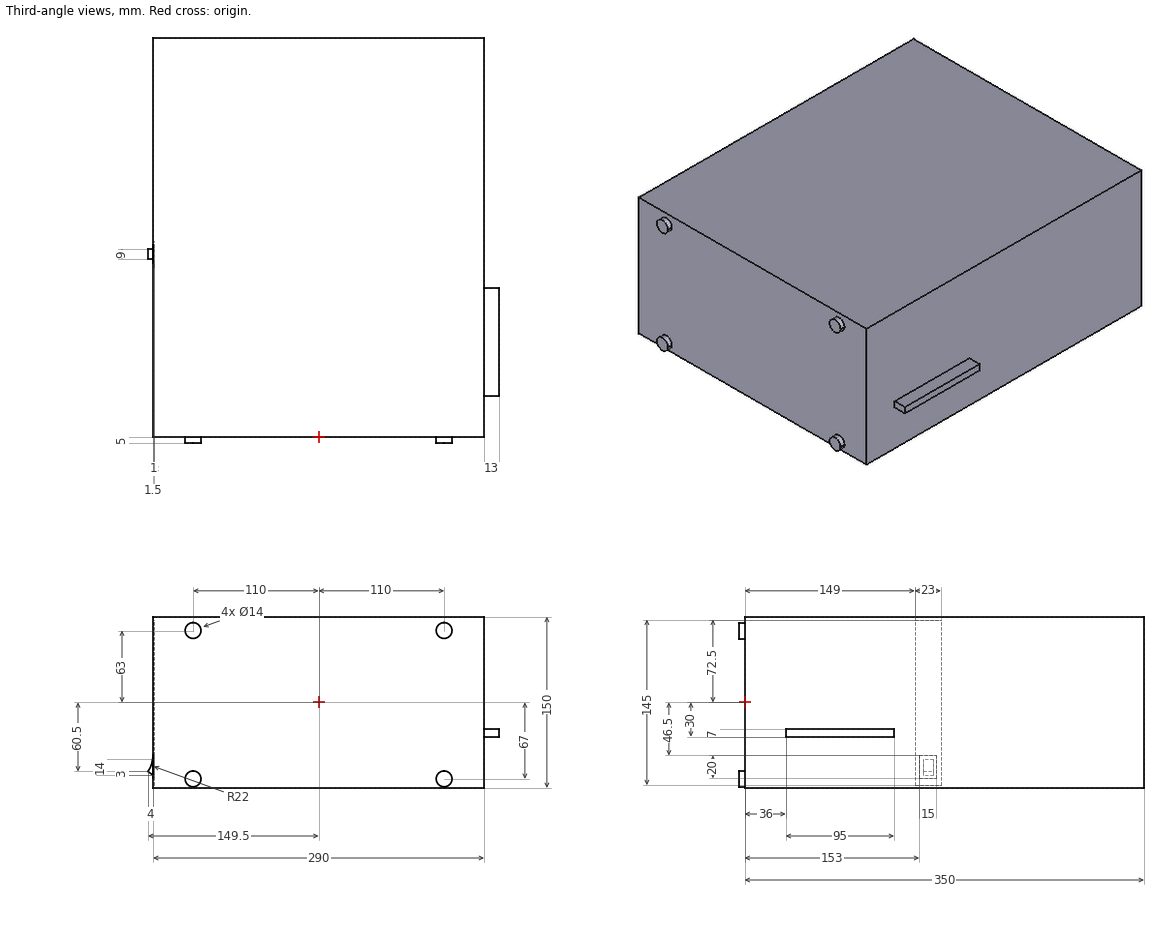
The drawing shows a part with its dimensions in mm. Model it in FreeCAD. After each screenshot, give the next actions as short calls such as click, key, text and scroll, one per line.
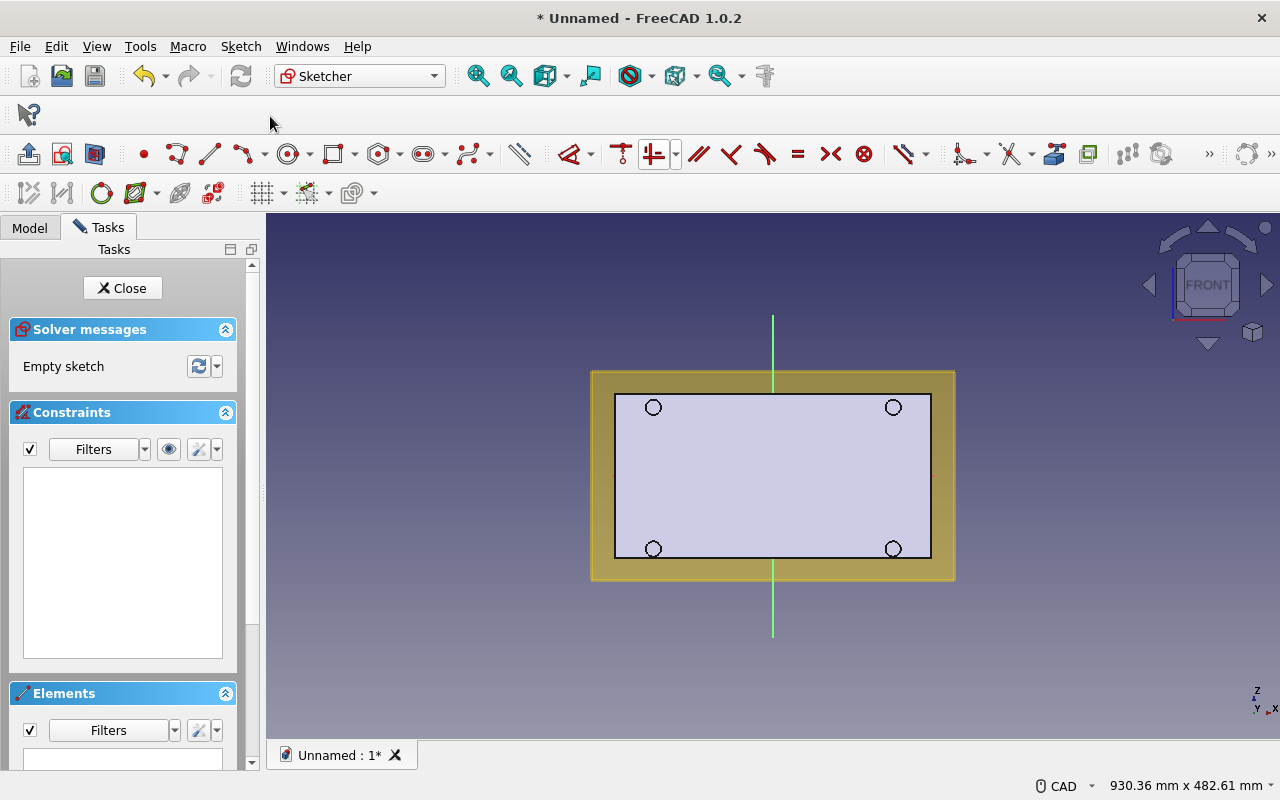
click(95, 154)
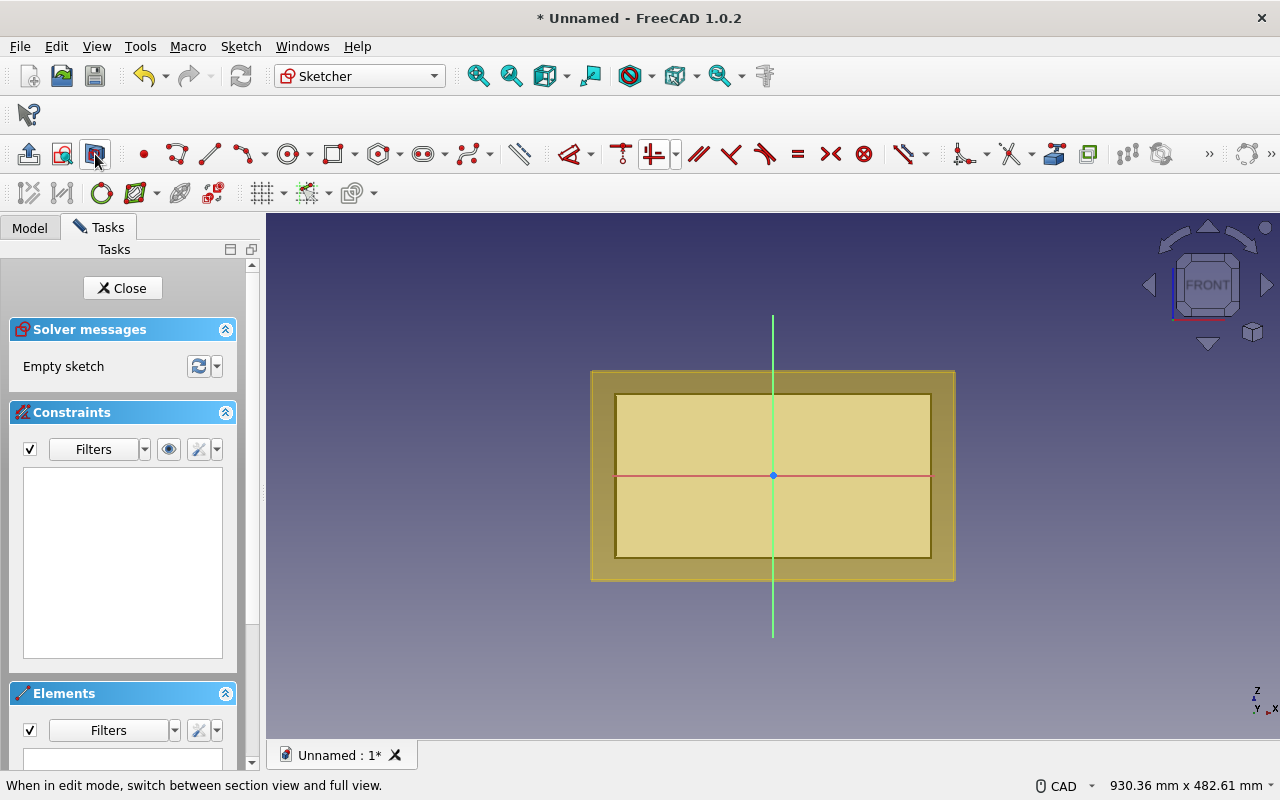
scroll(608, 541, up, 15)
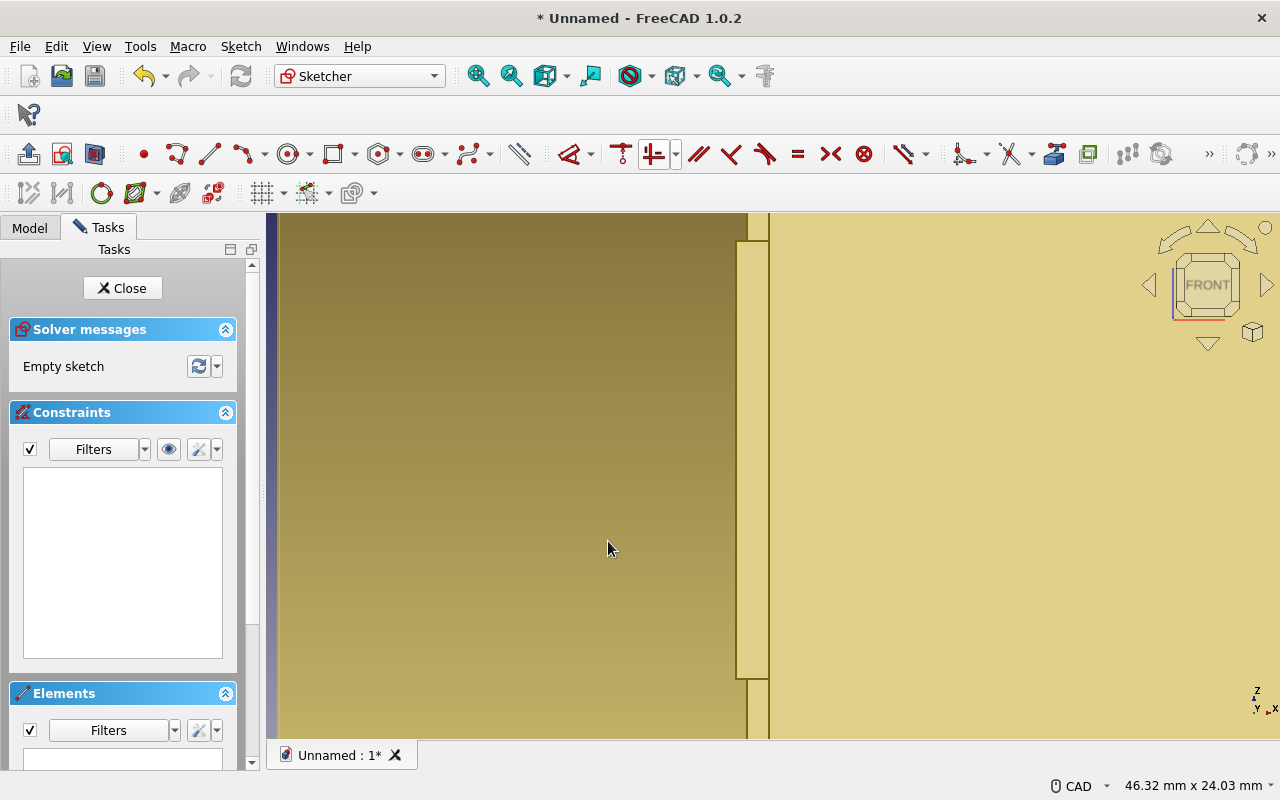
click(177, 154)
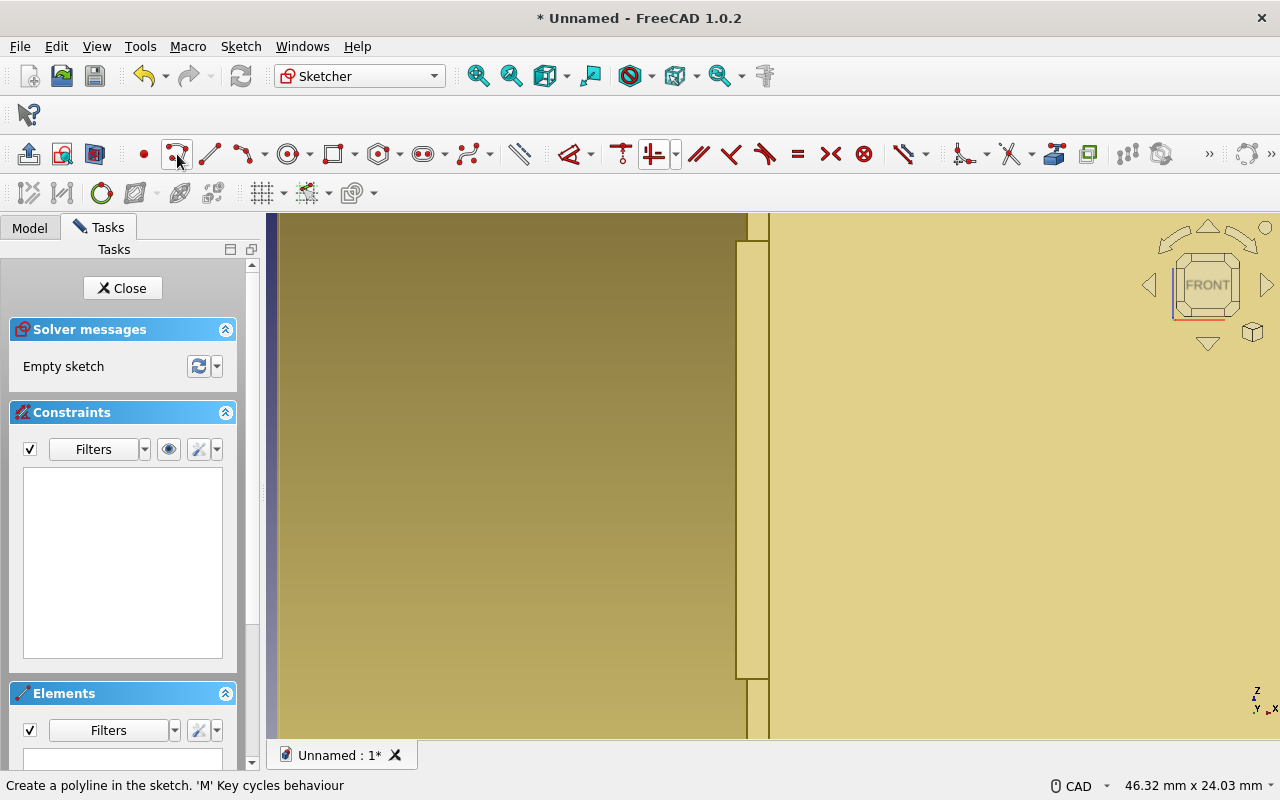
click(648, 548)
click(736, 614)
click(736, 307)
right_click(736, 307)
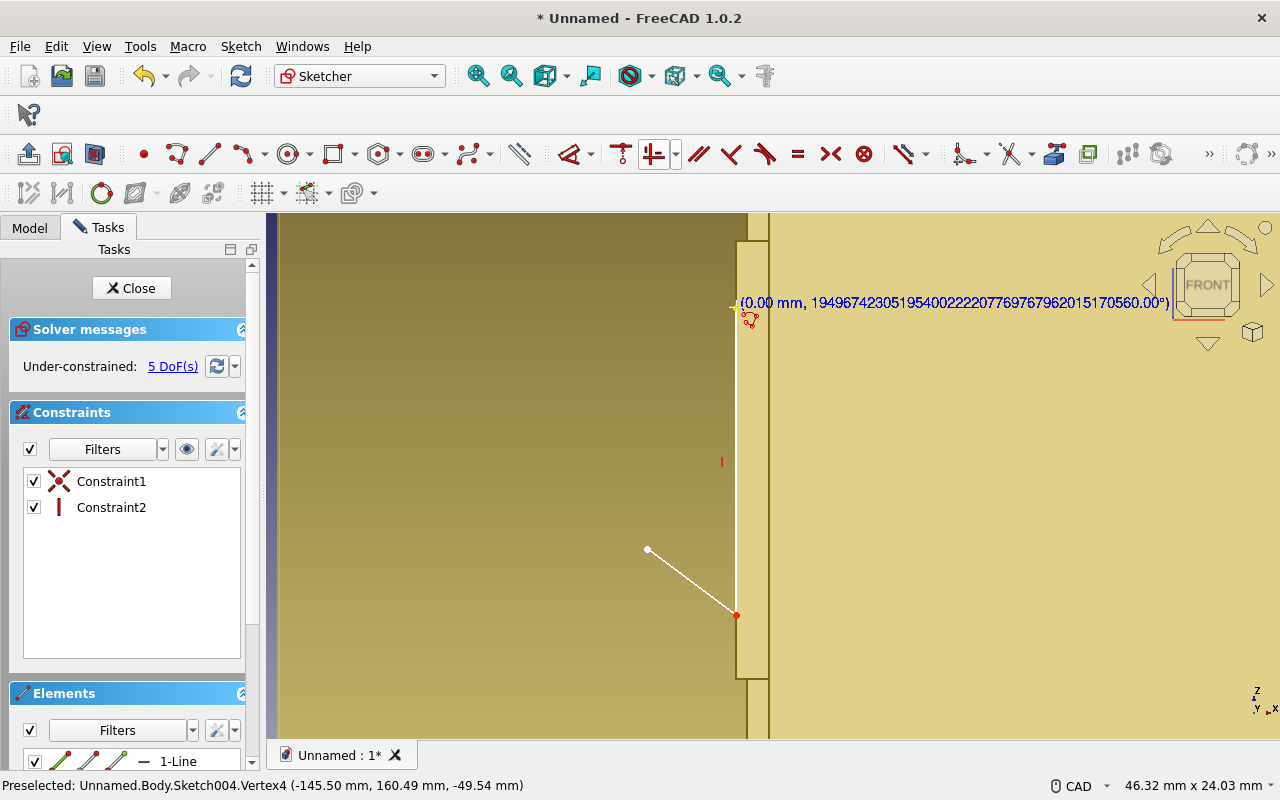
click(242, 154)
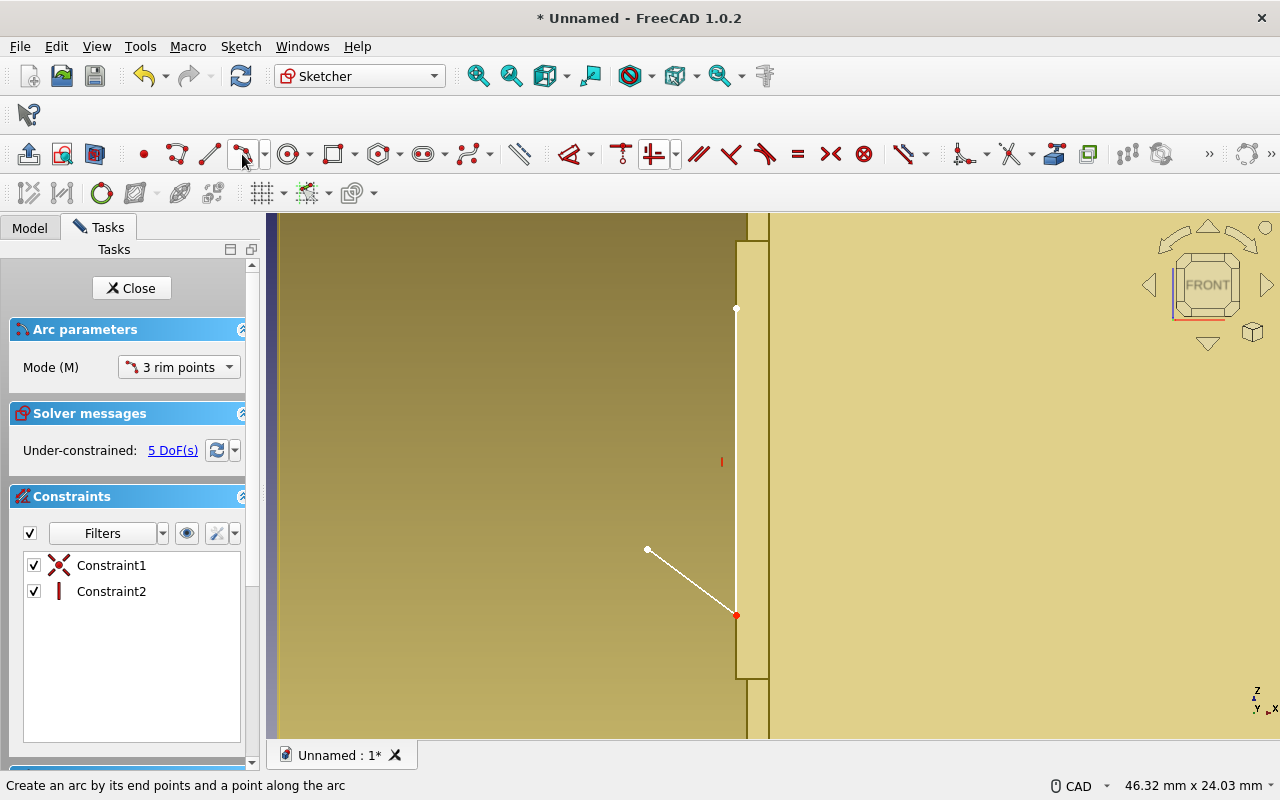
click(736, 308)
click(648, 549)
click(708, 433)
key(Escape)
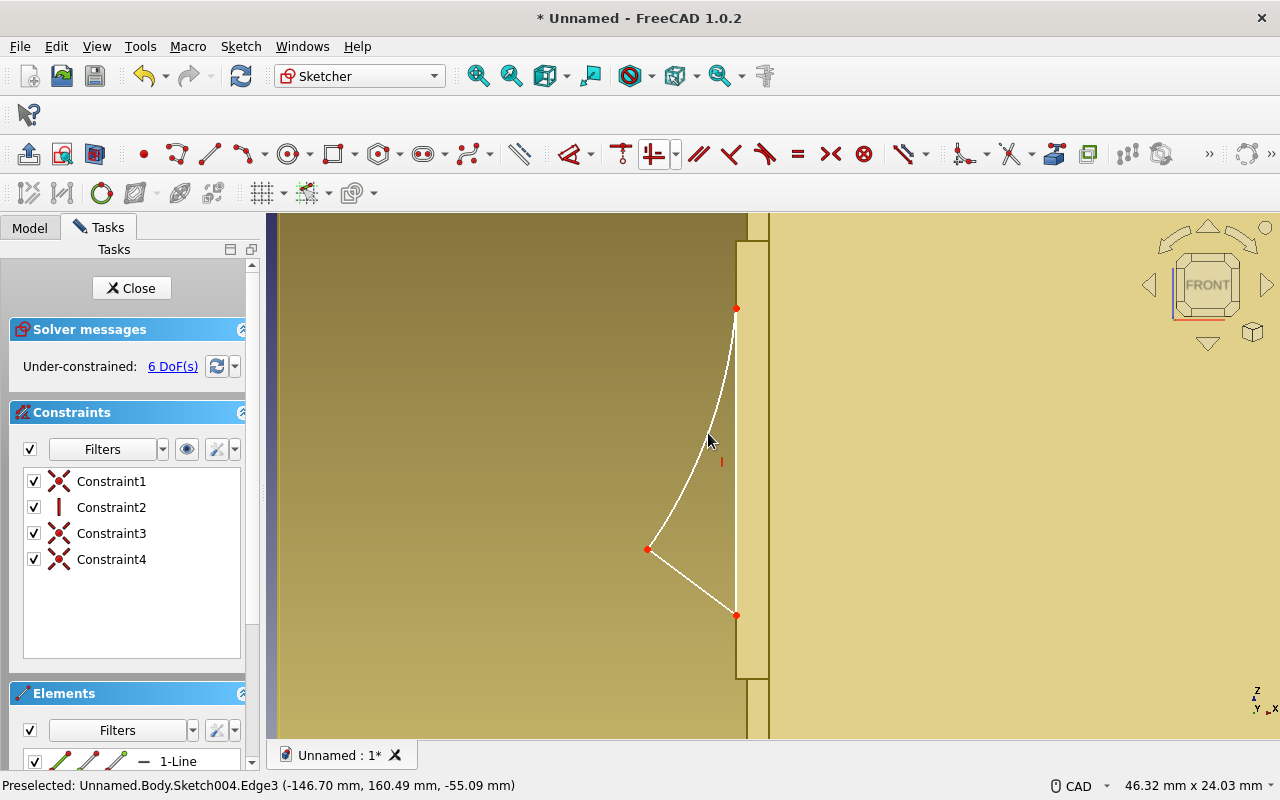
click(568, 154)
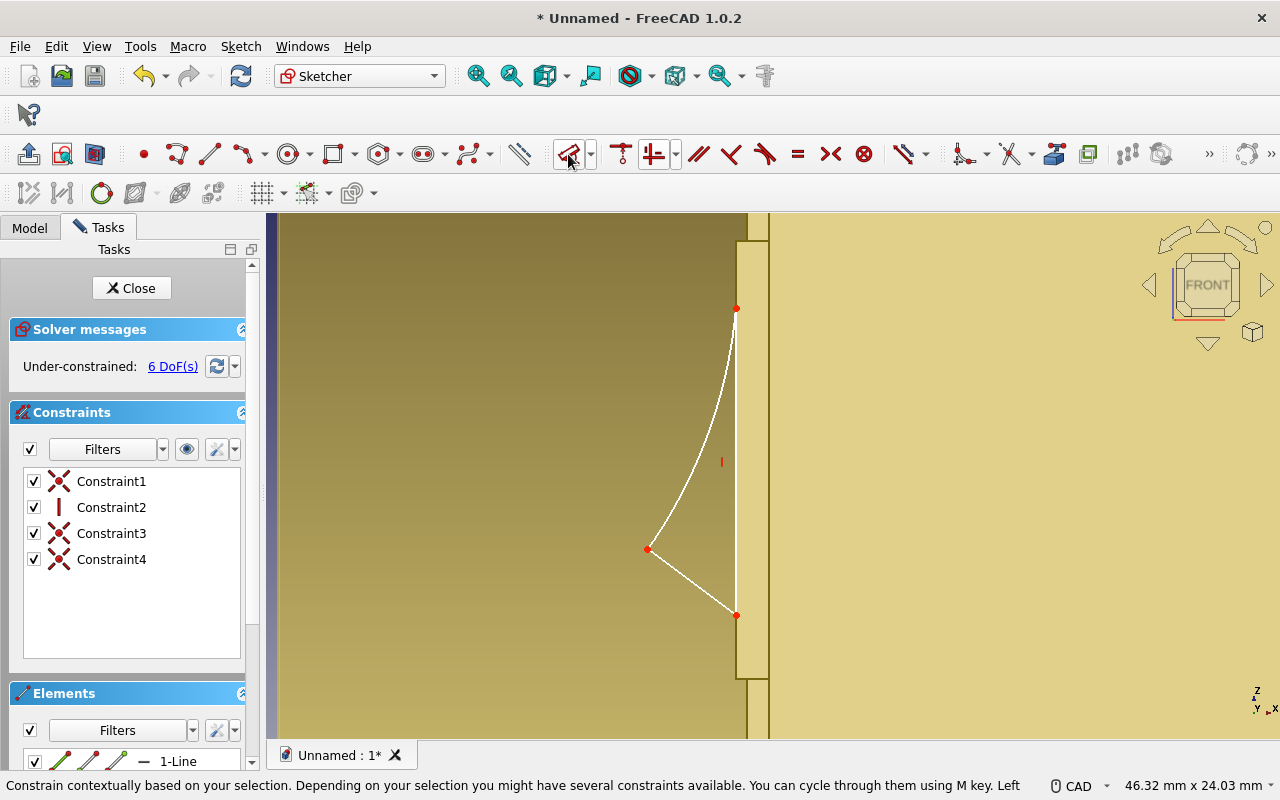
click(688, 482)
click(717, 496)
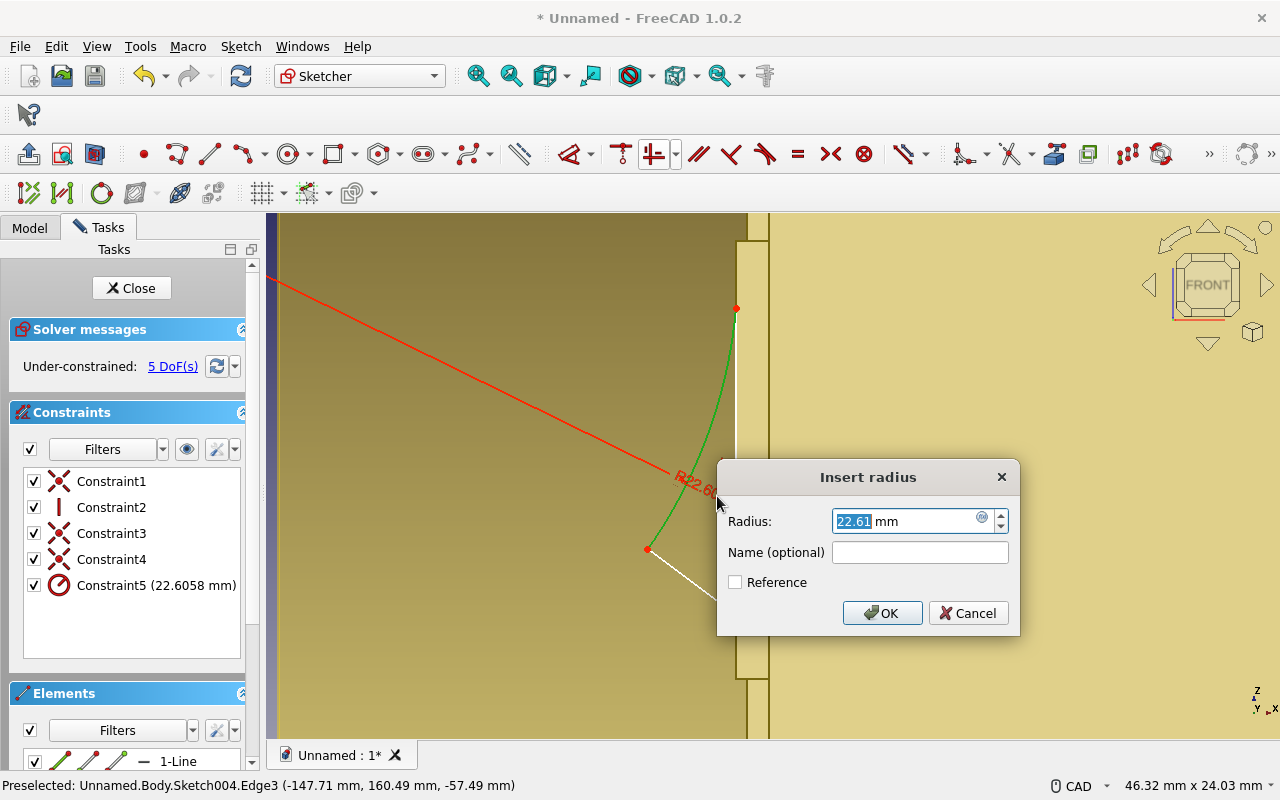
text(22)
key(Return)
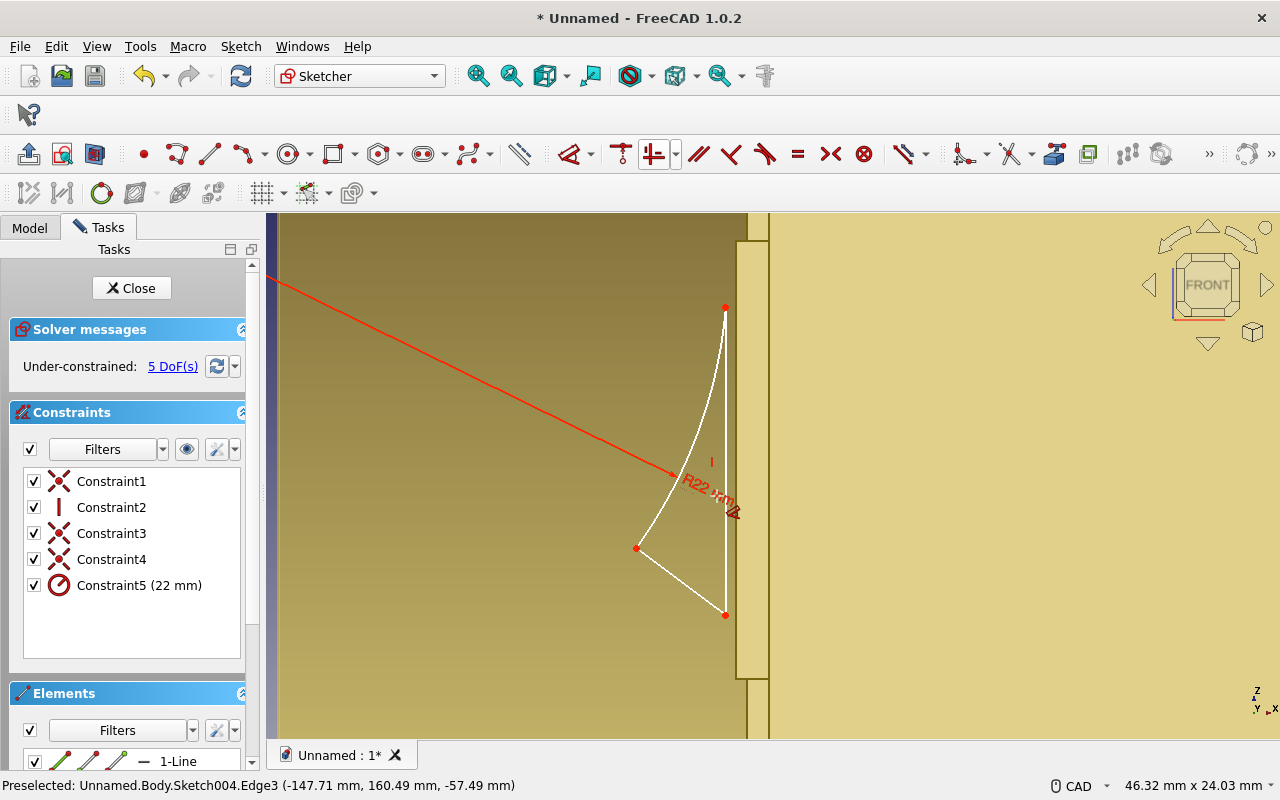
click(726, 523)
click(760, 461)